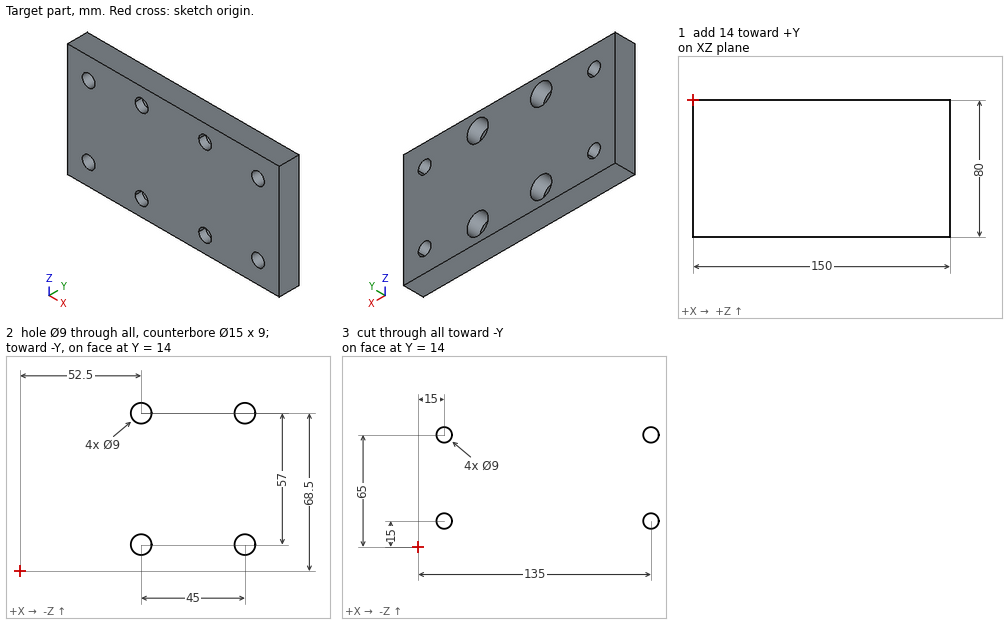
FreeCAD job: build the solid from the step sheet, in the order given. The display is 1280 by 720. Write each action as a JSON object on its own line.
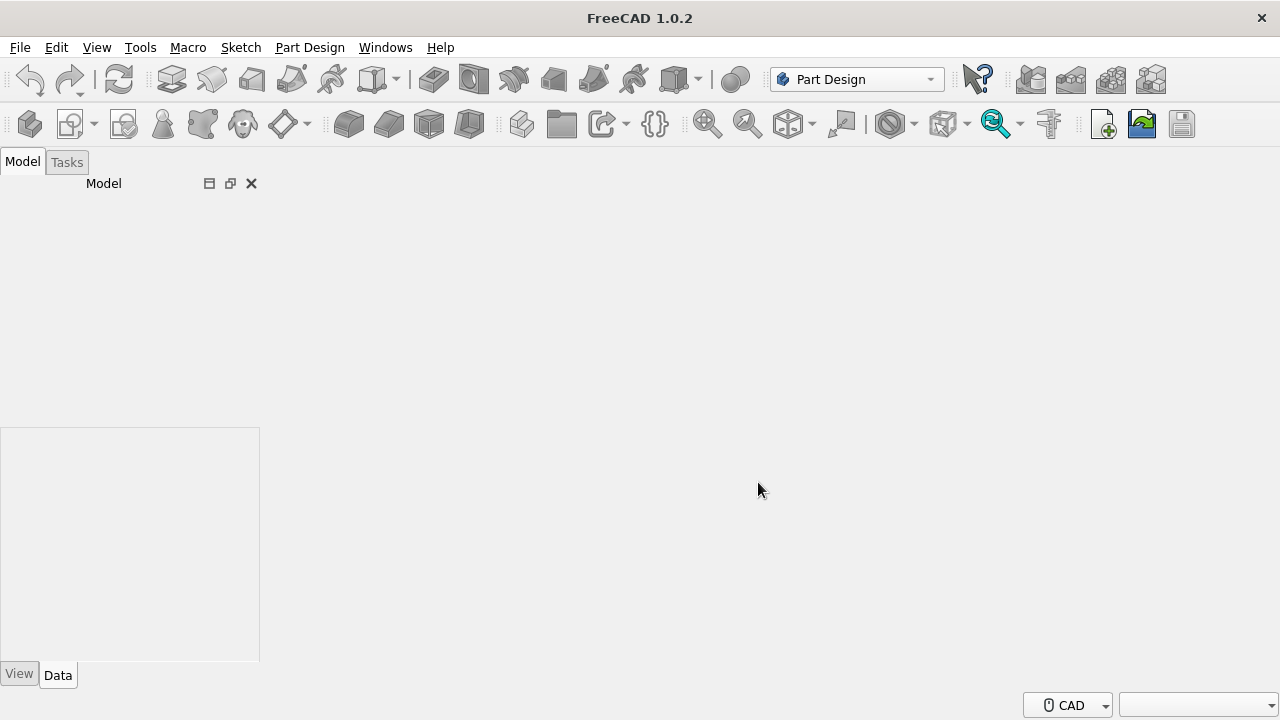
{"action": "left_click", "coordinate": [1102, 124]}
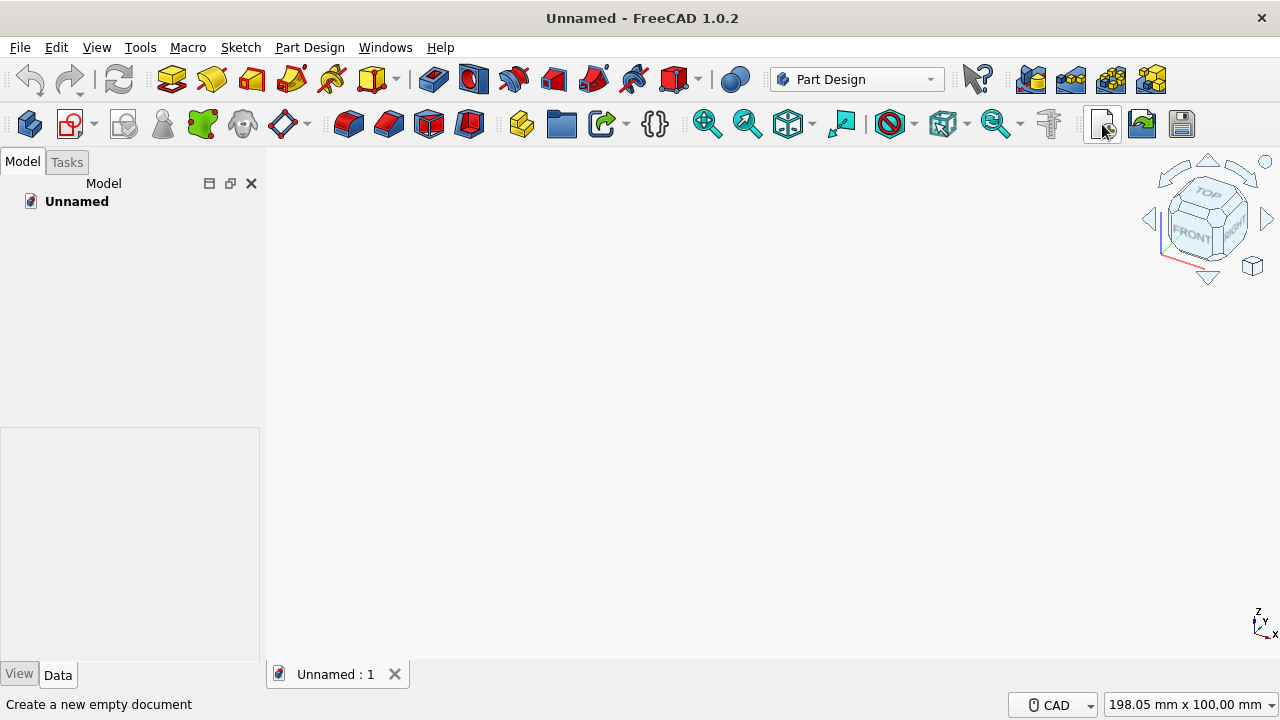
{"action": "left_click", "coordinate": [70, 124]}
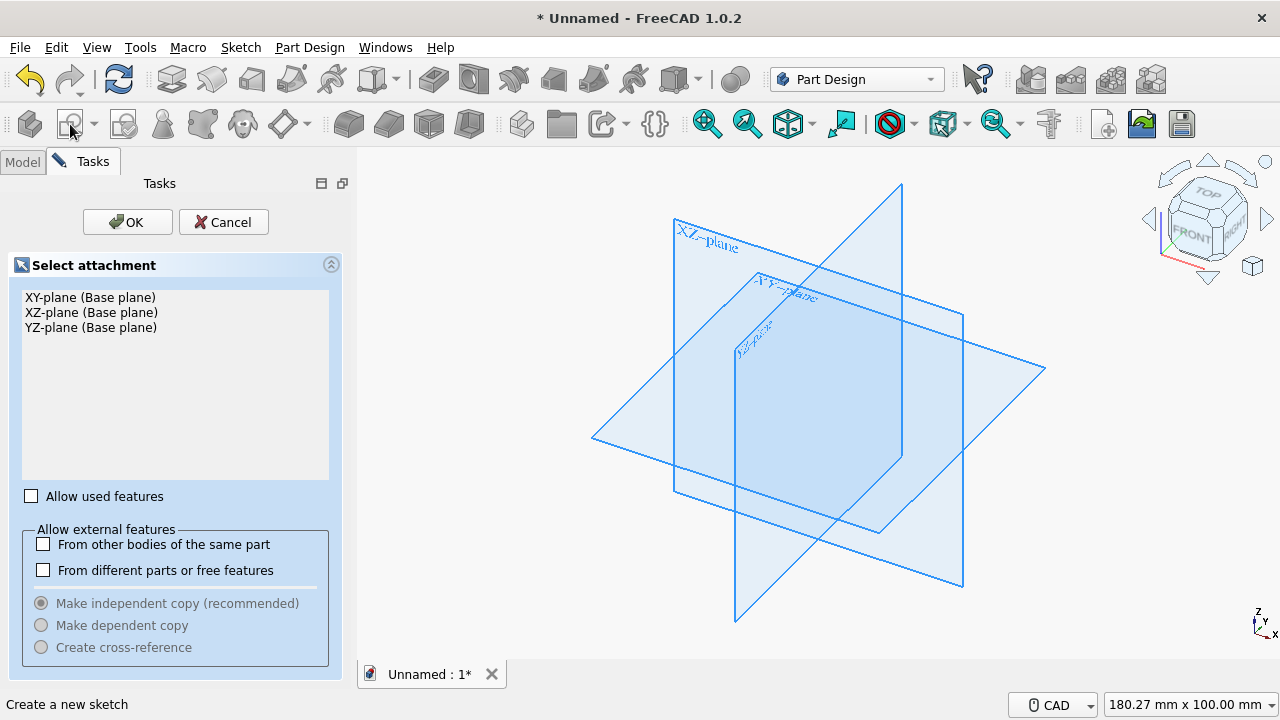
{"action": "left_click", "coordinate": [82, 312]}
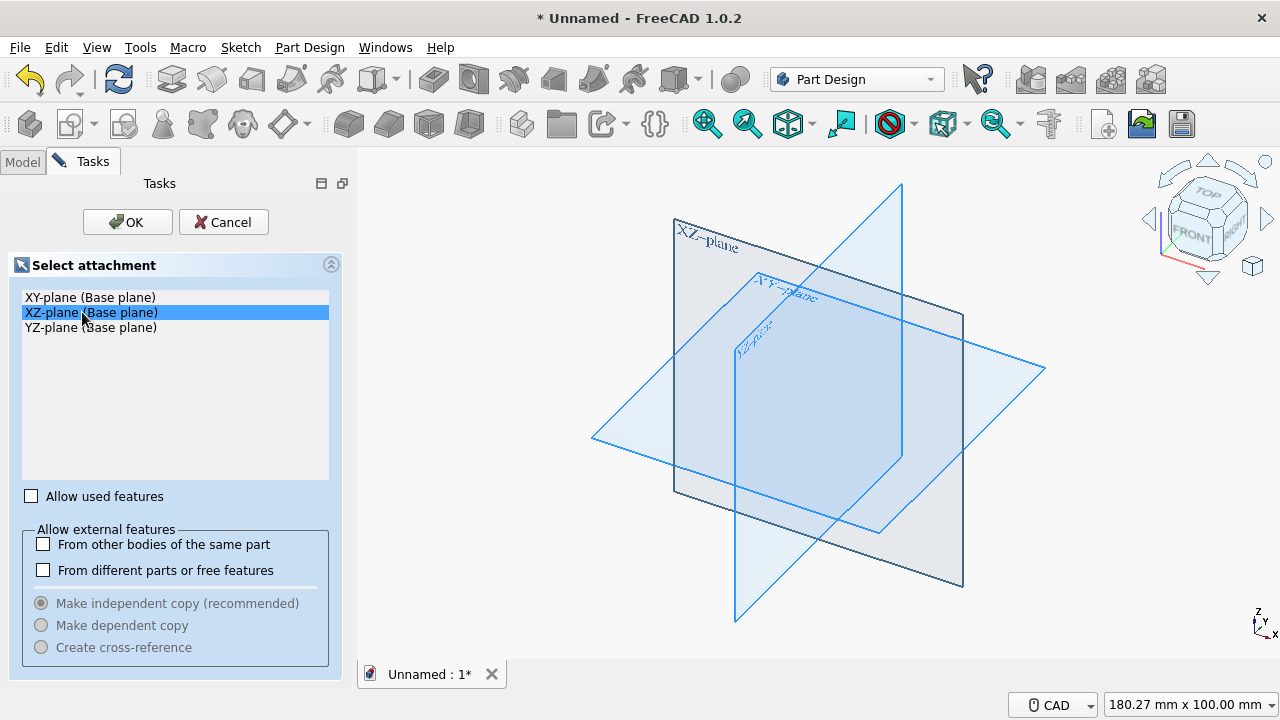
{"action": "left_click", "coordinate": [128, 222]}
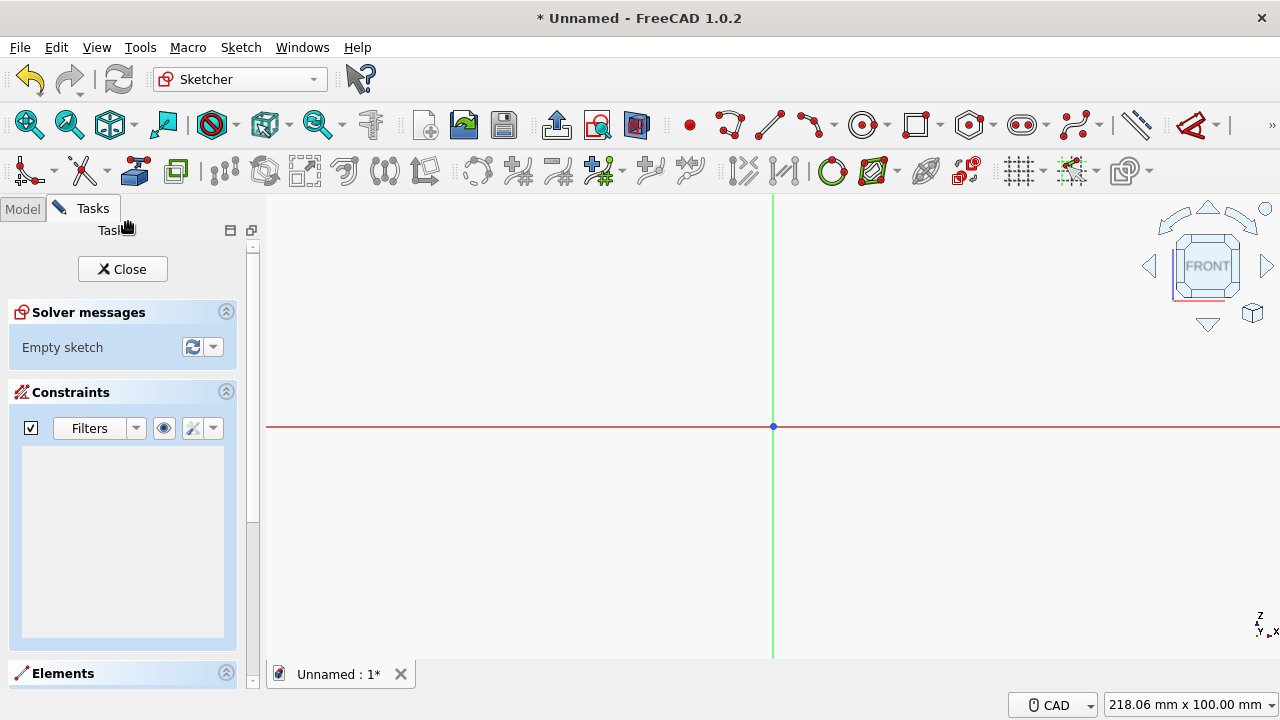
{"action": "scroll", "coordinate": [294, 222], "scroll_direction": "down", "scroll_amount": 3}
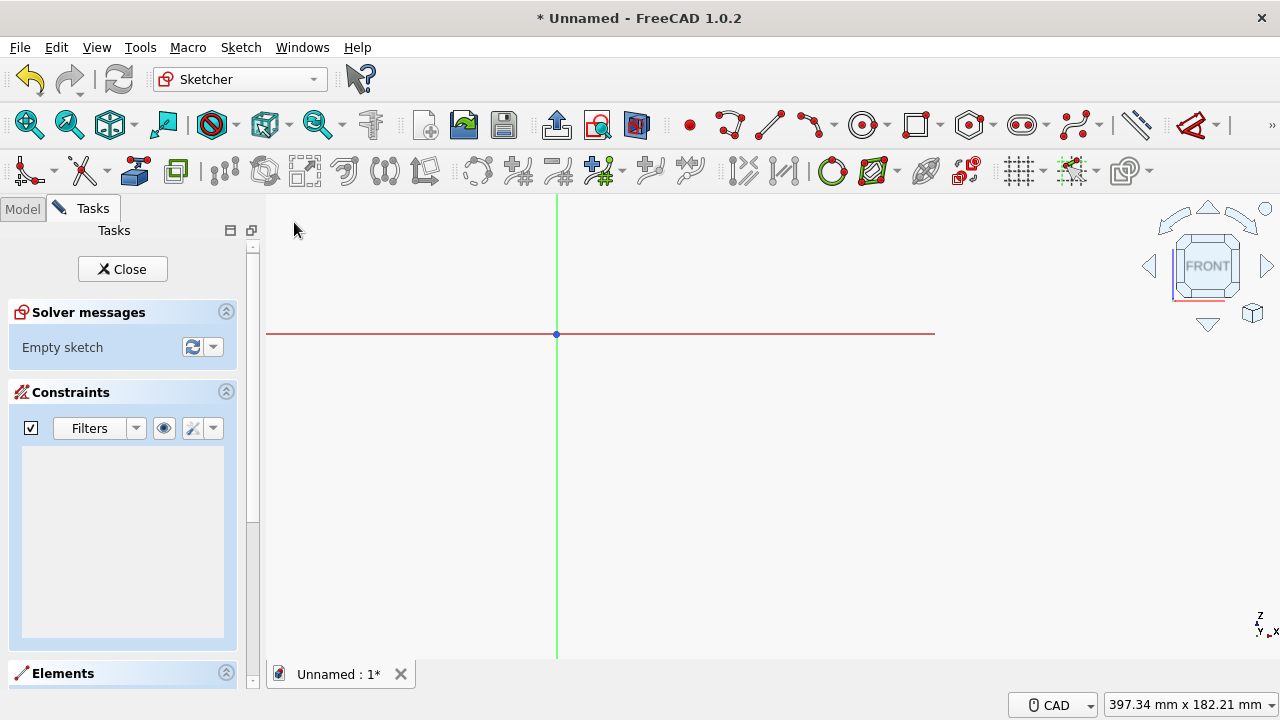
{"action": "scroll", "coordinate": [837, 456], "scroll_direction": "up", "scroll_amount": 2}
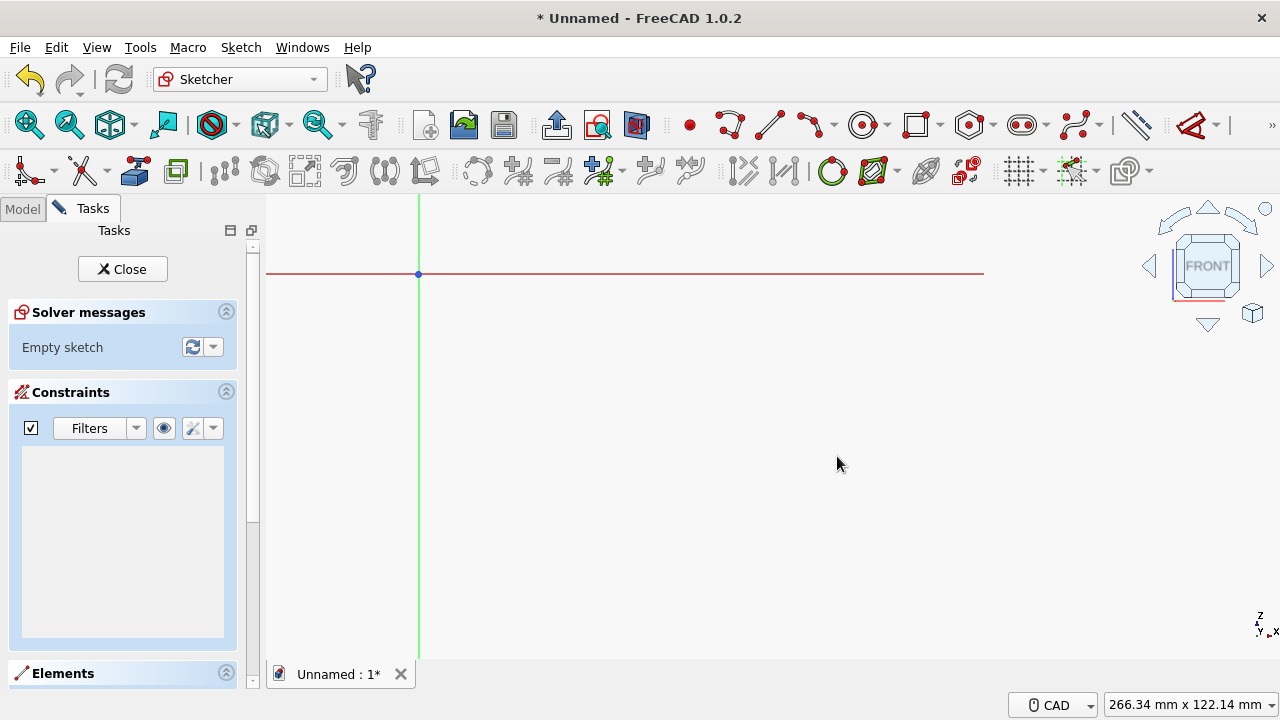
{"action": "left_click", "coordinate": [916, 126]}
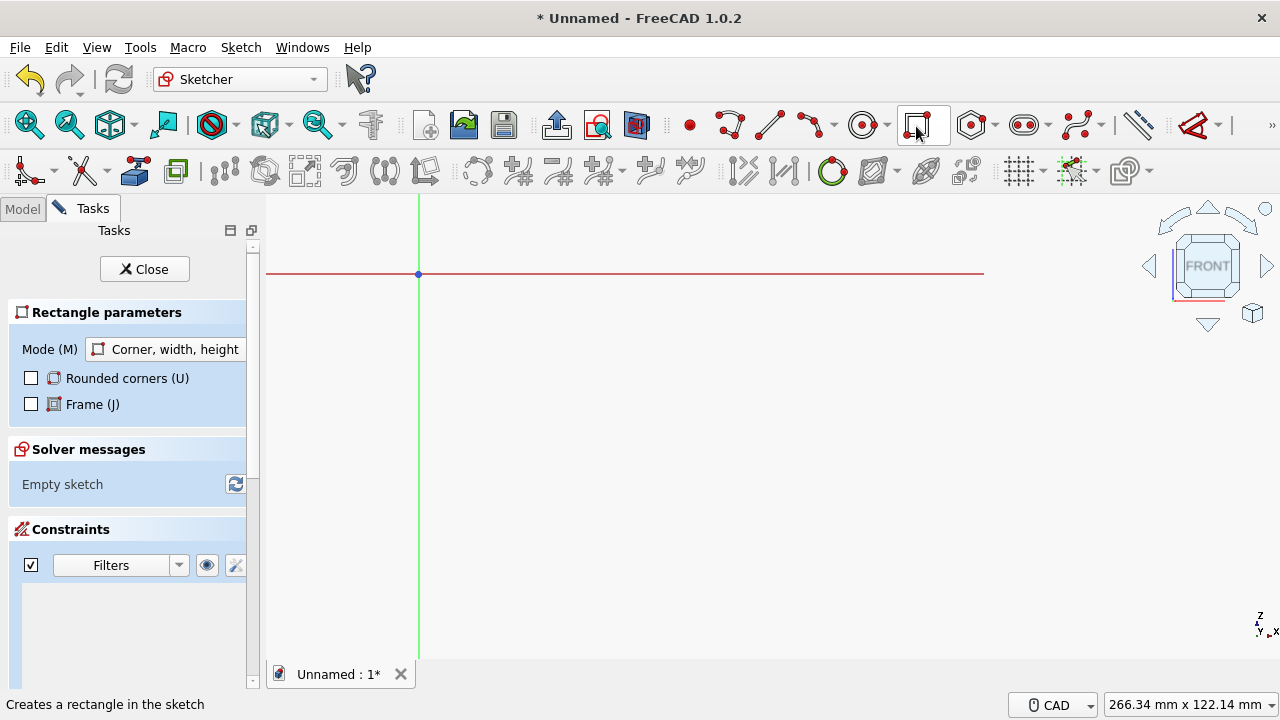
{"action": "left_click", "coordinate": [419, 274]}
{"action": "mouse_move", "coordinate": [990, 579]}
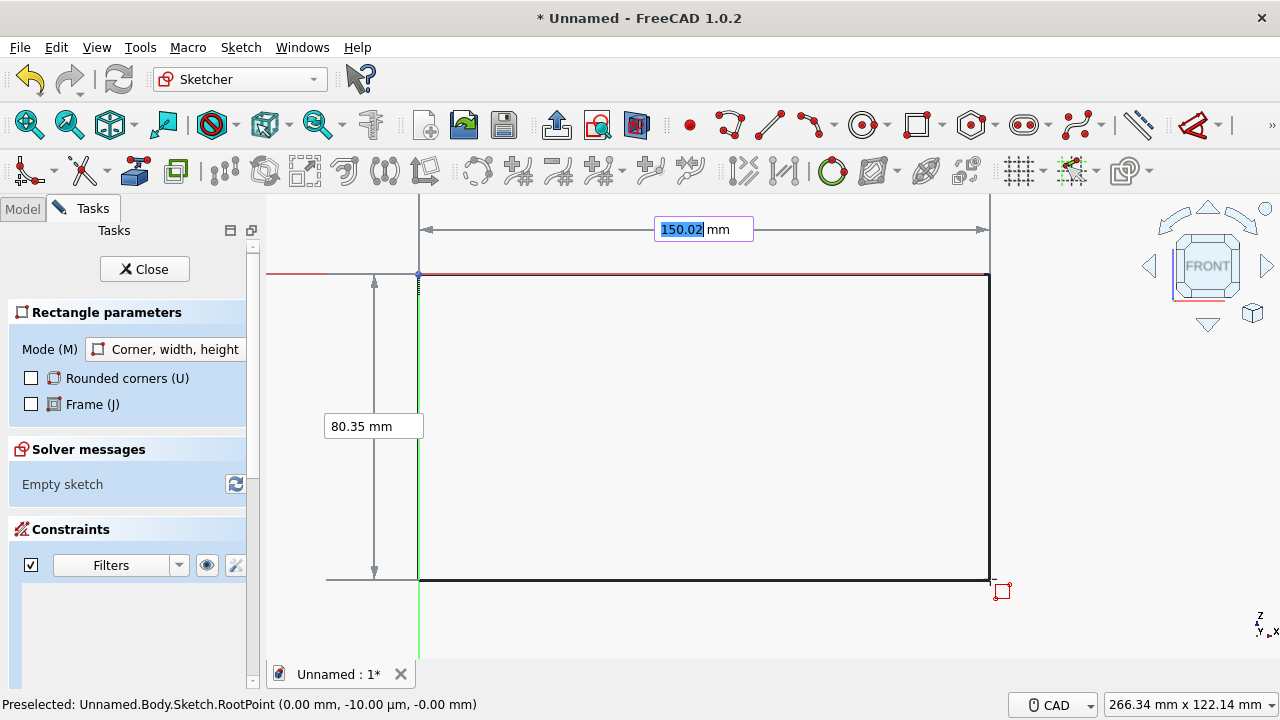
{"action": "type", "text": "150"}
{"action": "key", "text": "Tab"}
{"action": "type", "text": "80"}
{"action": "key", "text": "Return"}
{"action": "key", "text": "Escape"}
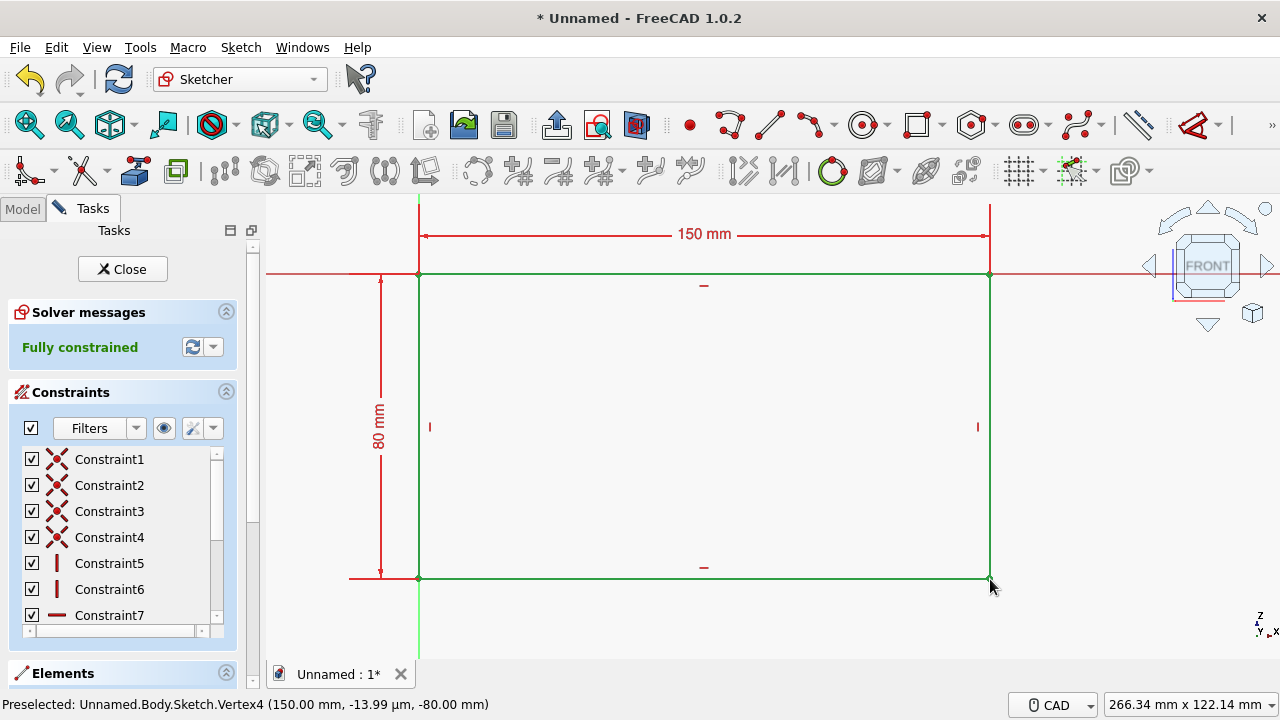
{"action": "left_click", "coordinate": [123, 269]}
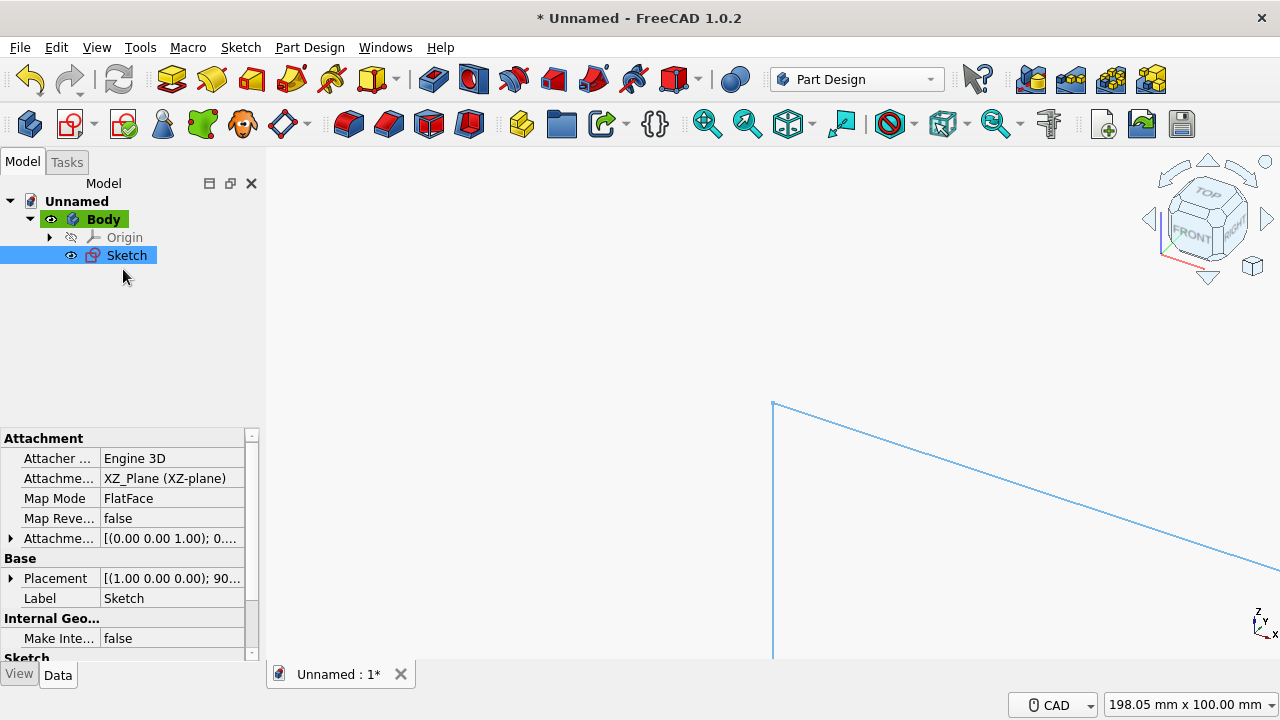
{"action": "left_click", "coordinate": [172, 80]}